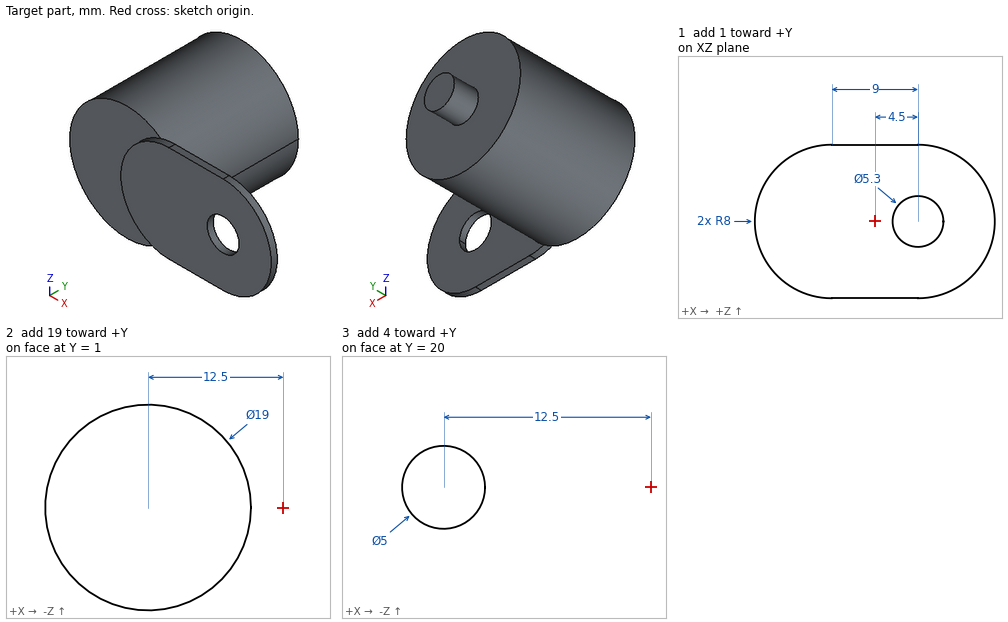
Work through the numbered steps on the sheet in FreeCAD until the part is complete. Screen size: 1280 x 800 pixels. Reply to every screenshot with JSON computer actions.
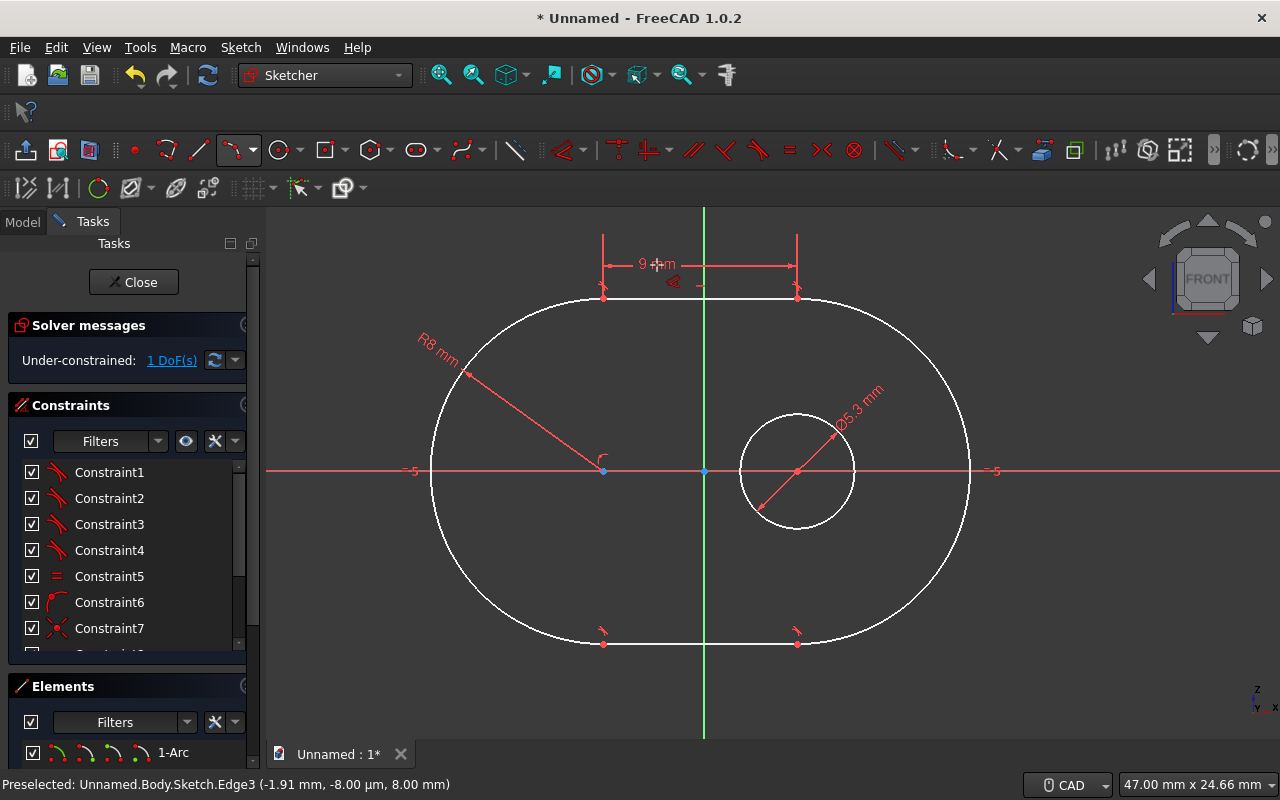
{"action": "left_click", "coordinate": [797, 471]}
{"action": "left_click", "coordinate": [729, 505]}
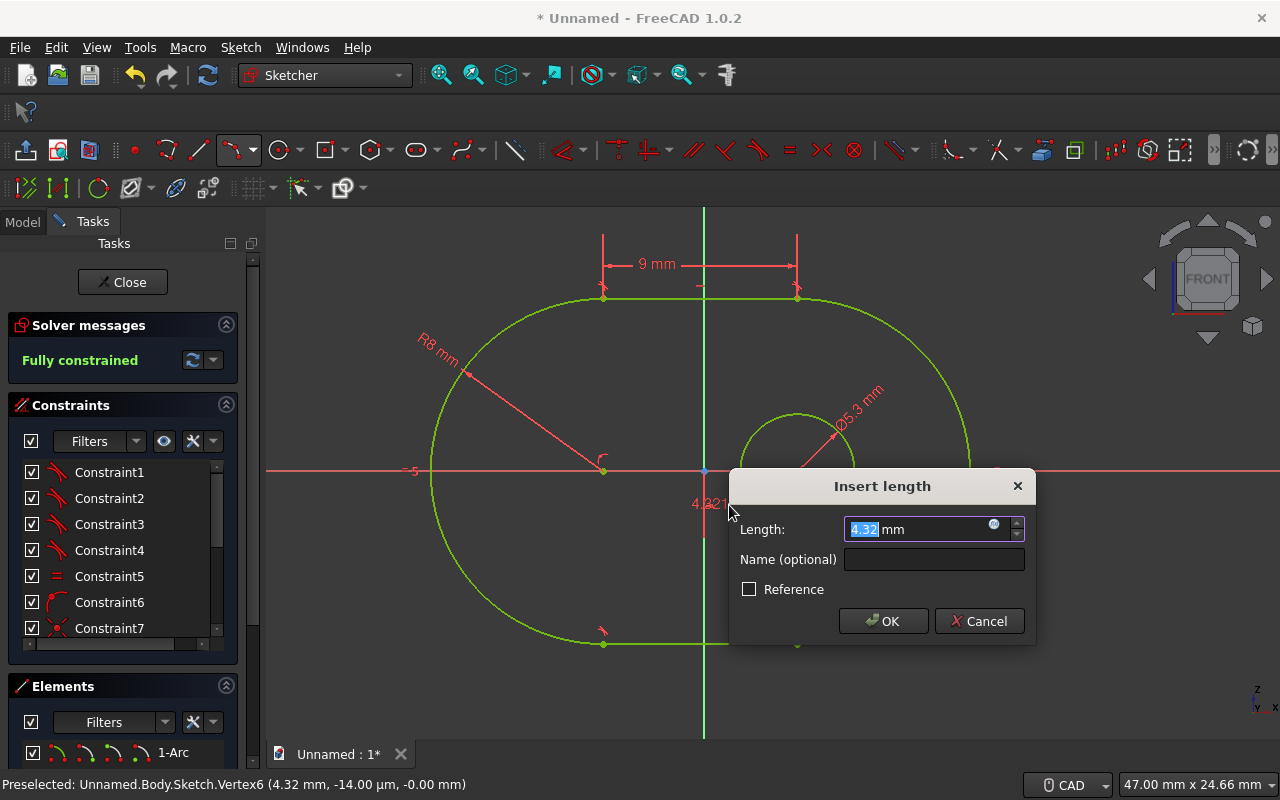
{"action": "type", "text": "4.5"}
{"action": "key", "text": "Return"}
{"action": "key", "text": "Escape"}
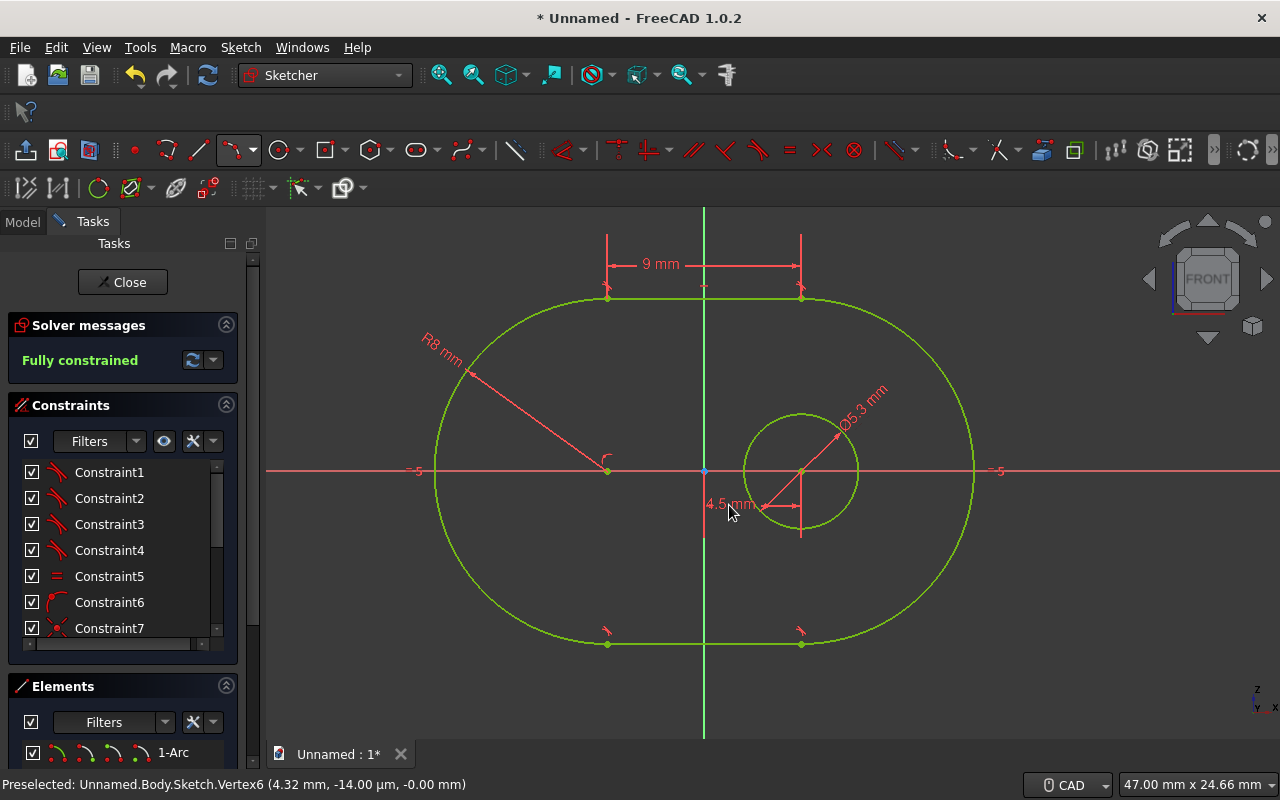
{"action": "left_click", "coordinate": [123, 282]}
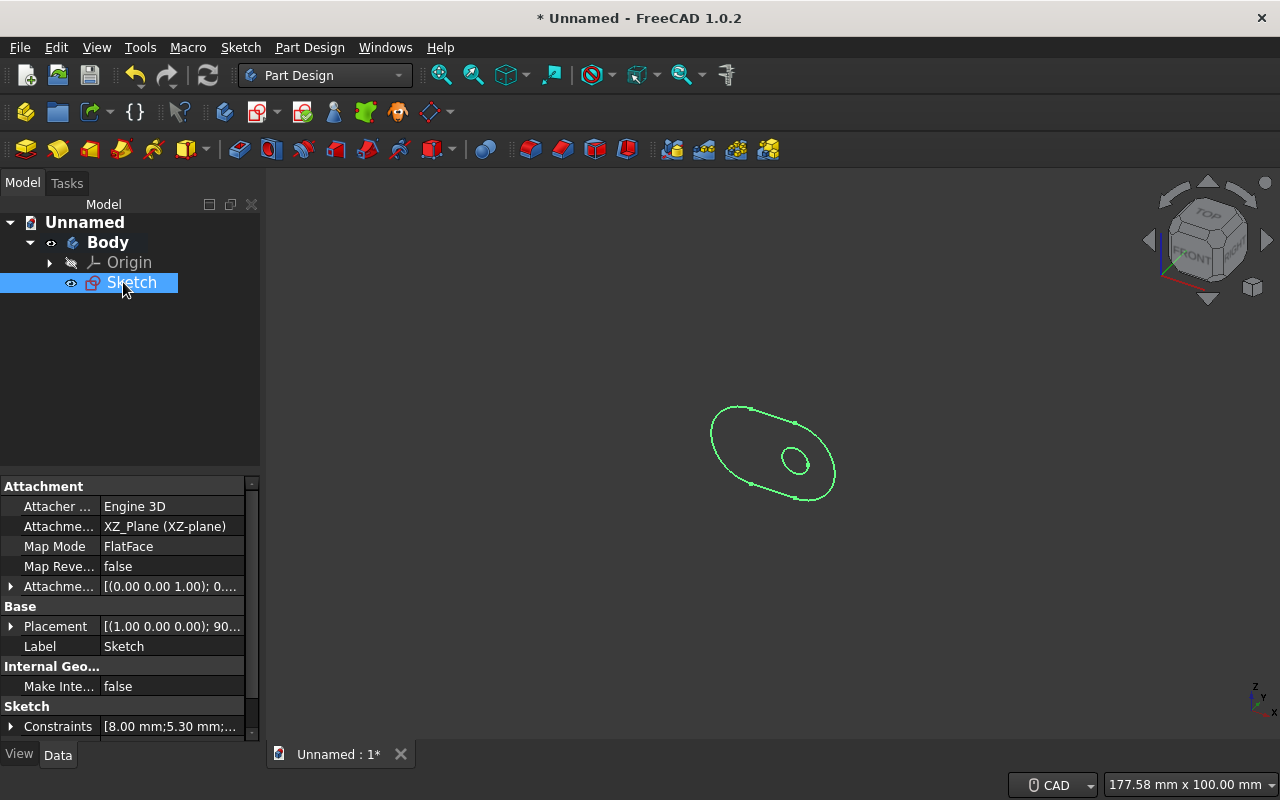
{"action": "left_click", "coordinate": [26, 150]}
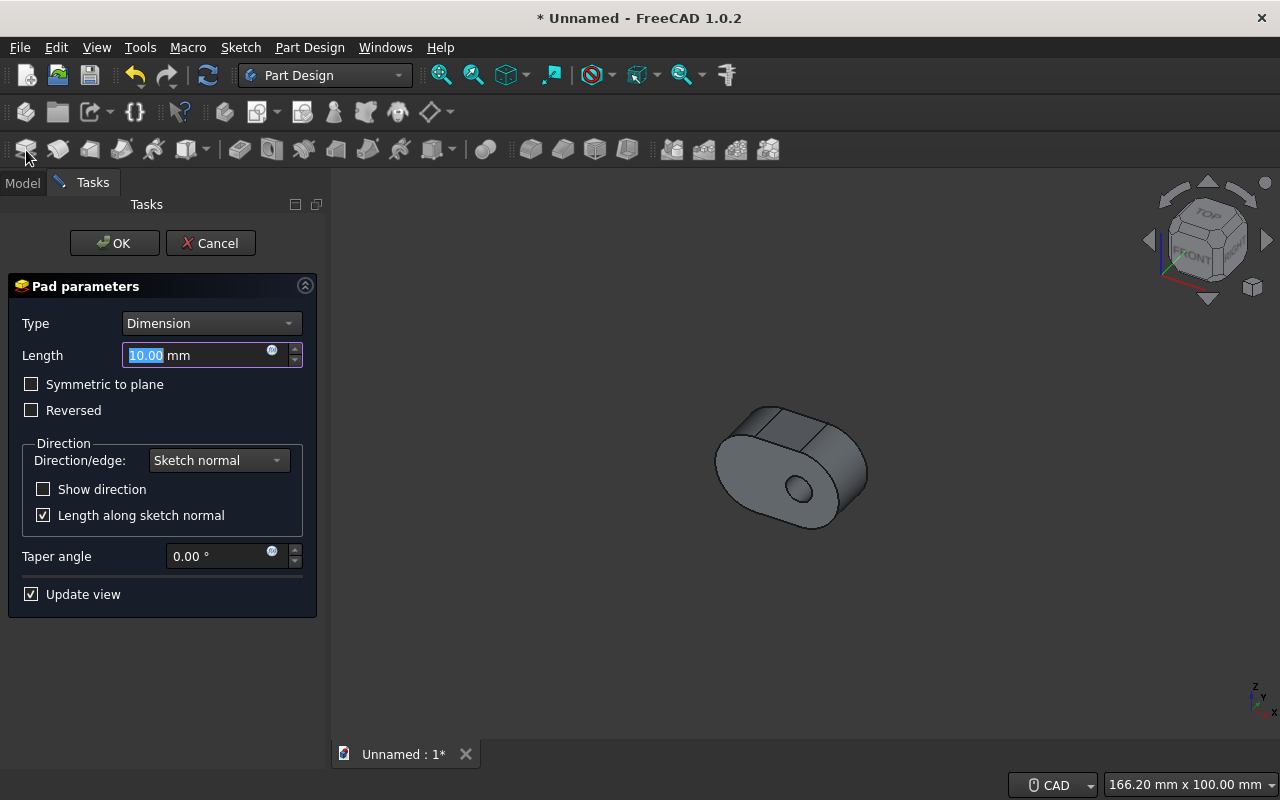
{"action": "type", "text": "1"}
{"action": "key", "text": "Tab"}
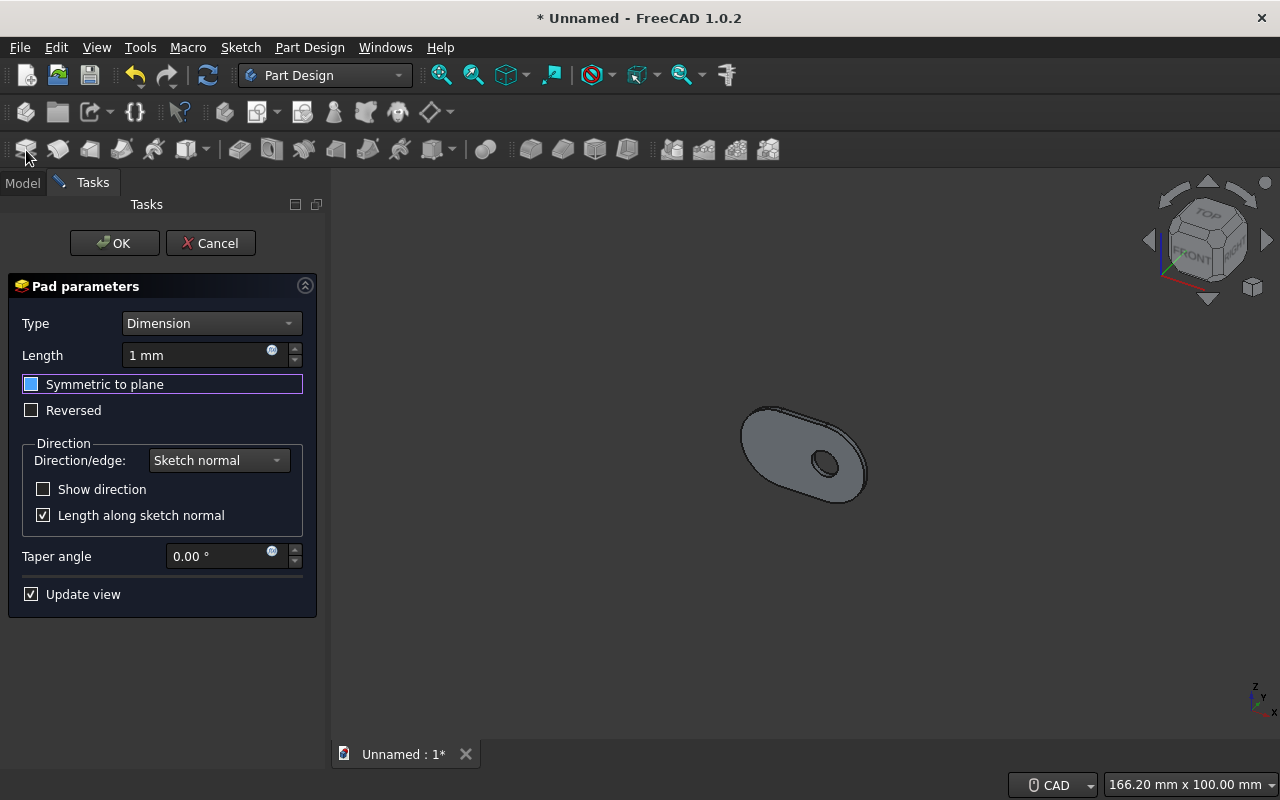
{"action": "left_click", "coordinate": [30, 410]}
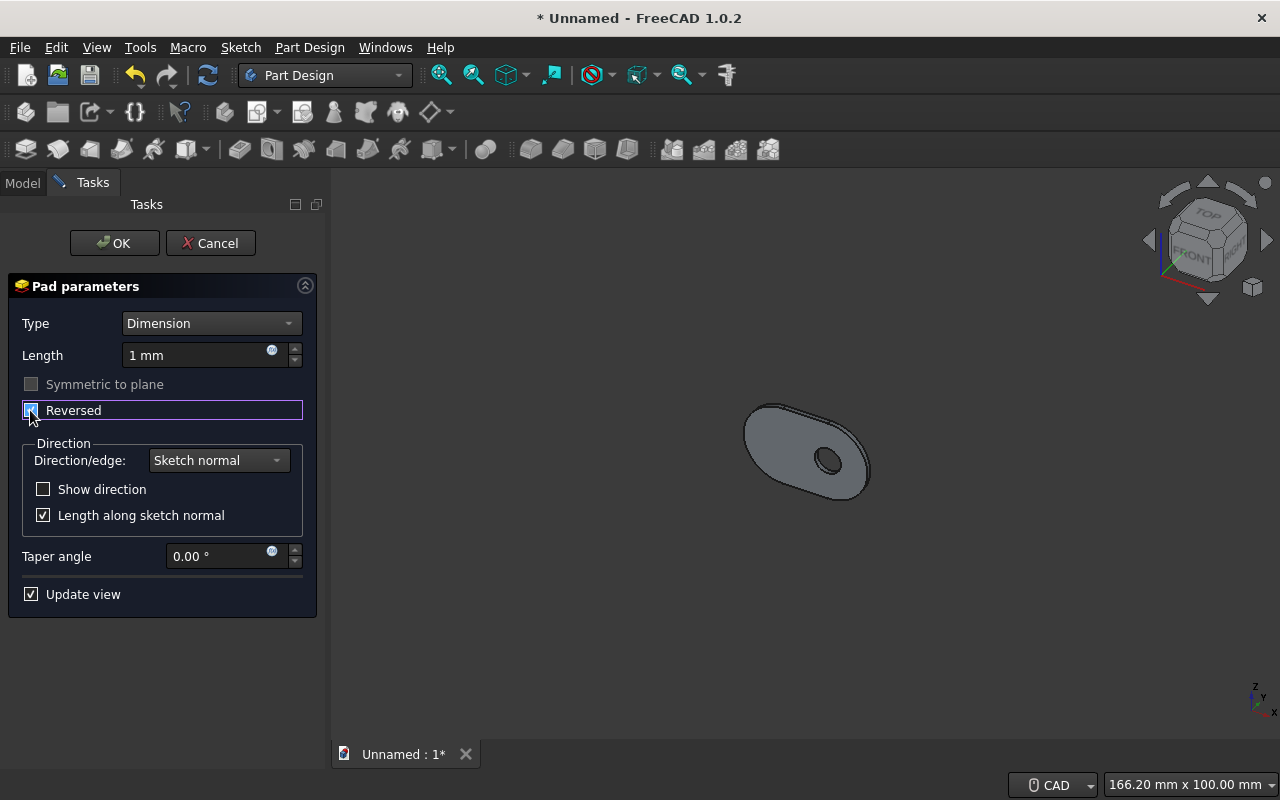
{"action": "left_click", "coordinate": [115, 243]}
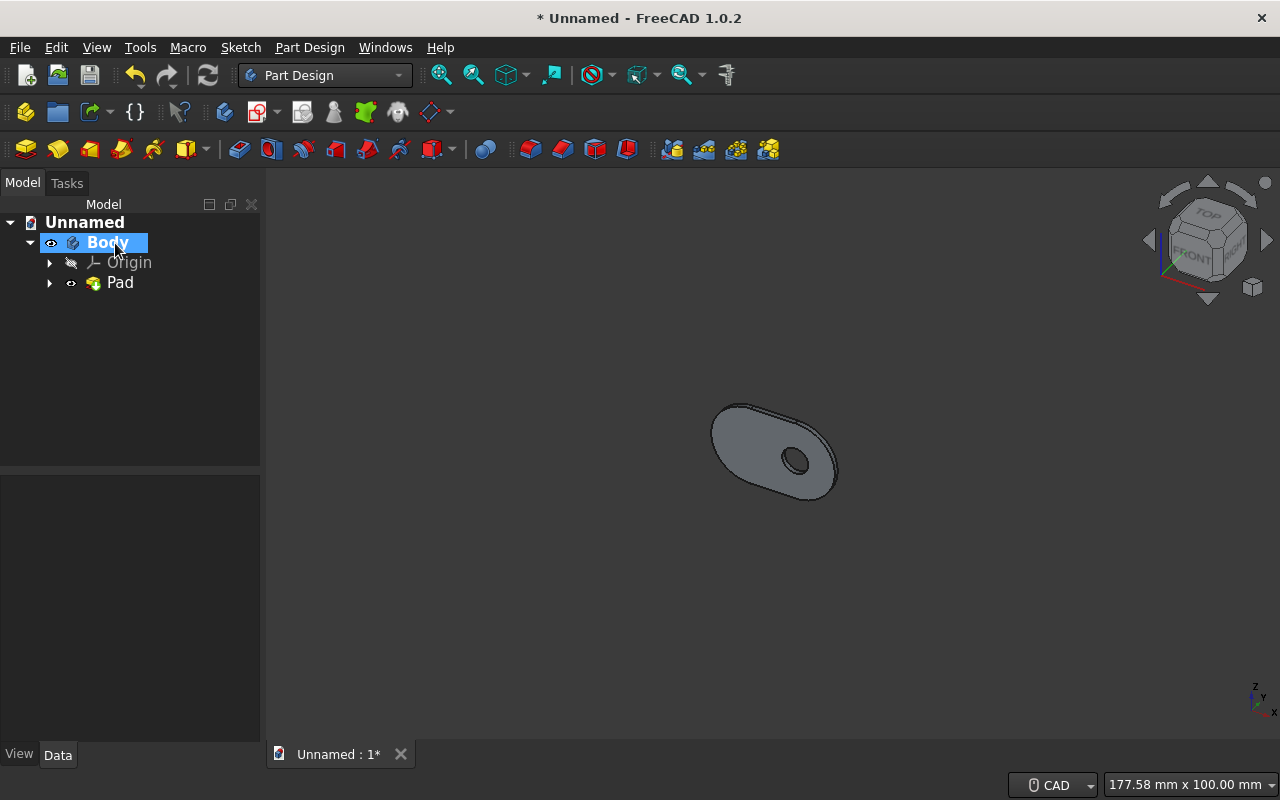
{"action": "left_click", "coordinate": [442, 76]}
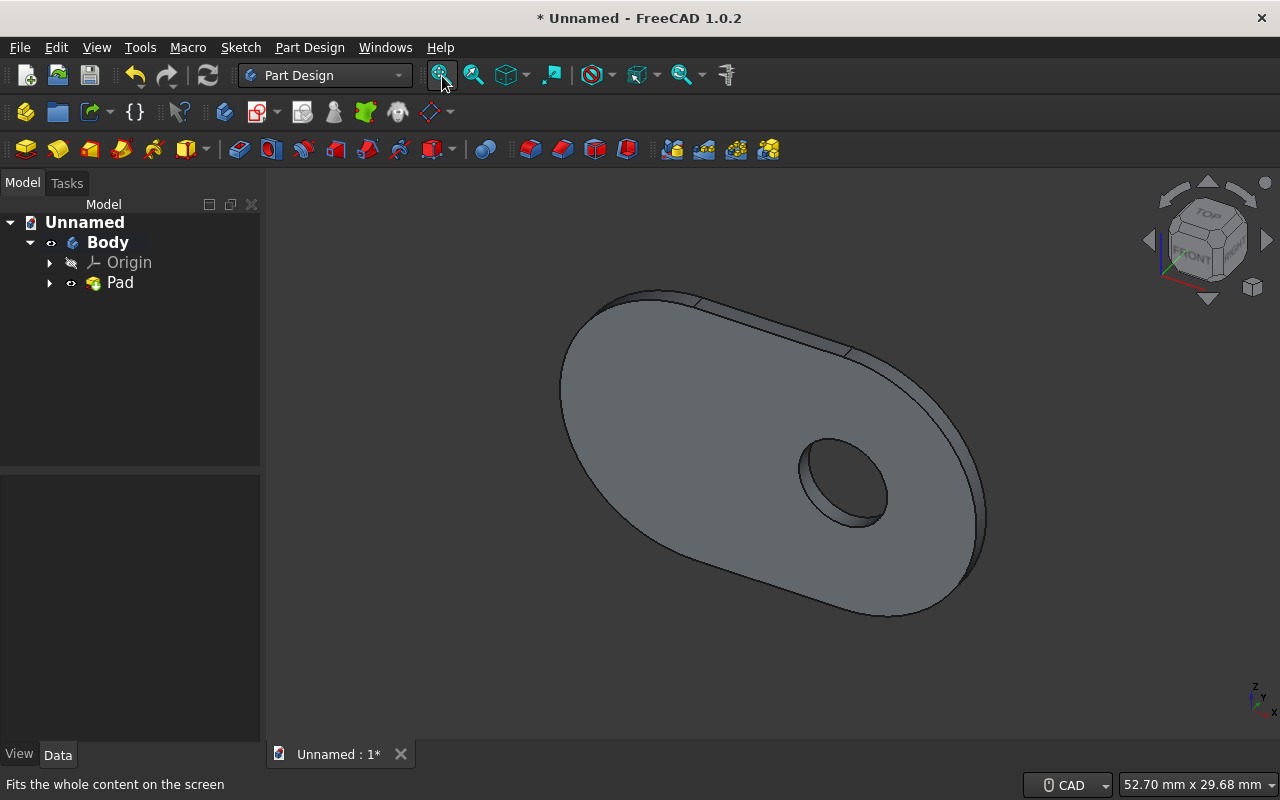
{"action": "key", "text": "4"}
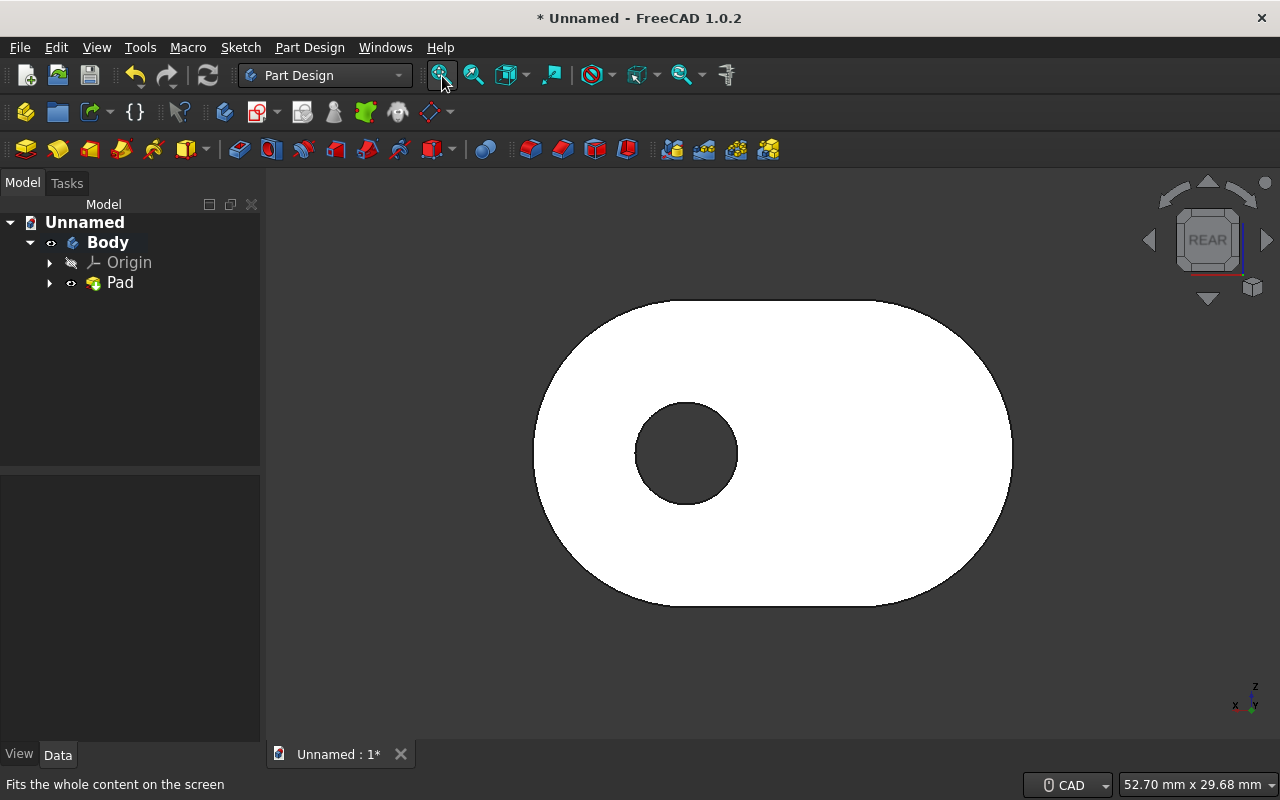
{"action": "left_click", "coordinate": [842, 409]}